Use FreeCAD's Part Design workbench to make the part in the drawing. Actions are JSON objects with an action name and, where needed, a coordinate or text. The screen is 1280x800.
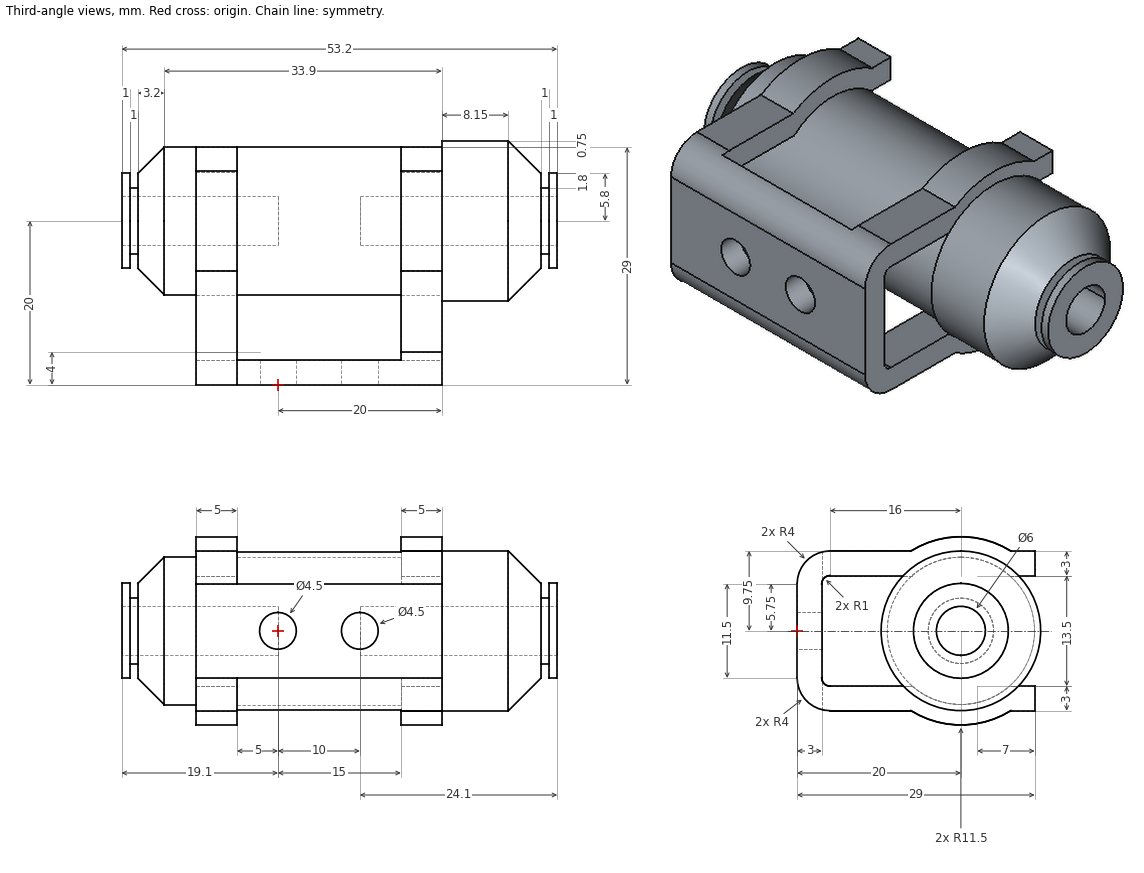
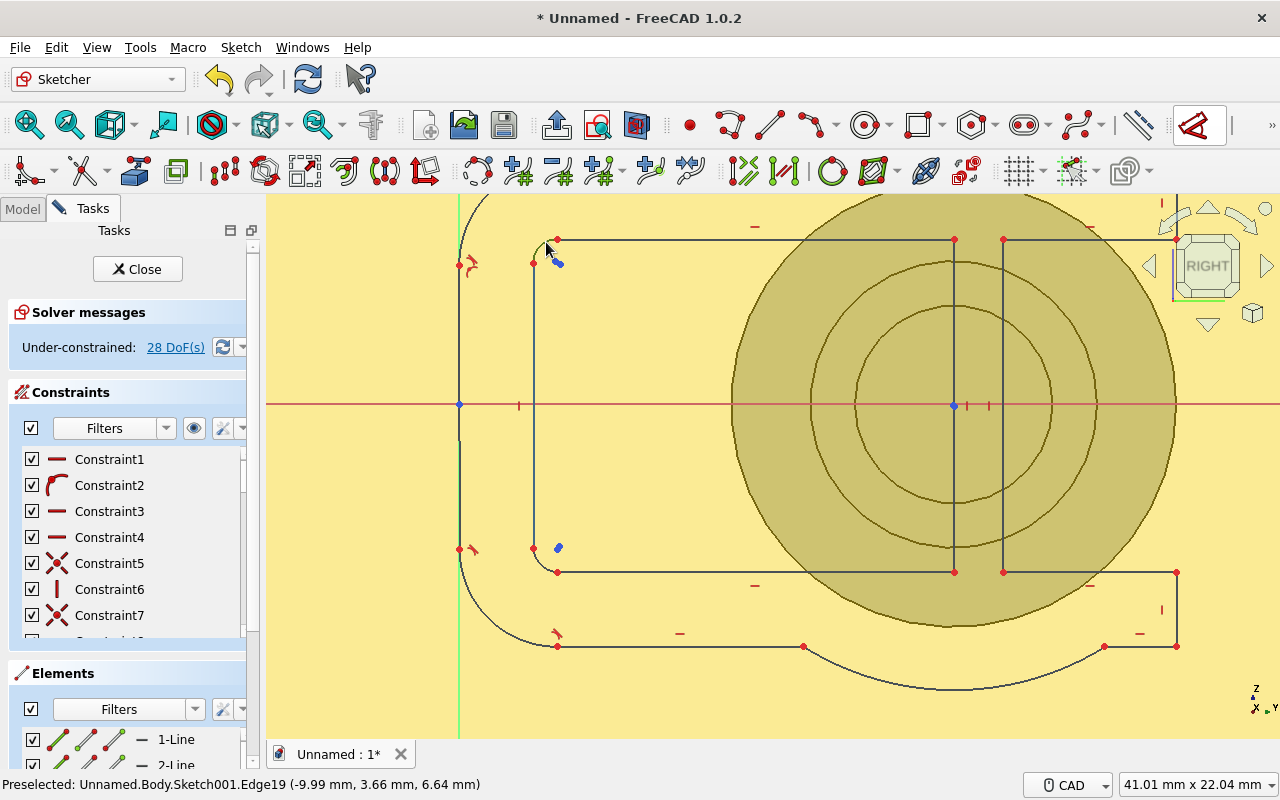
{"action": "key", "text": "t"}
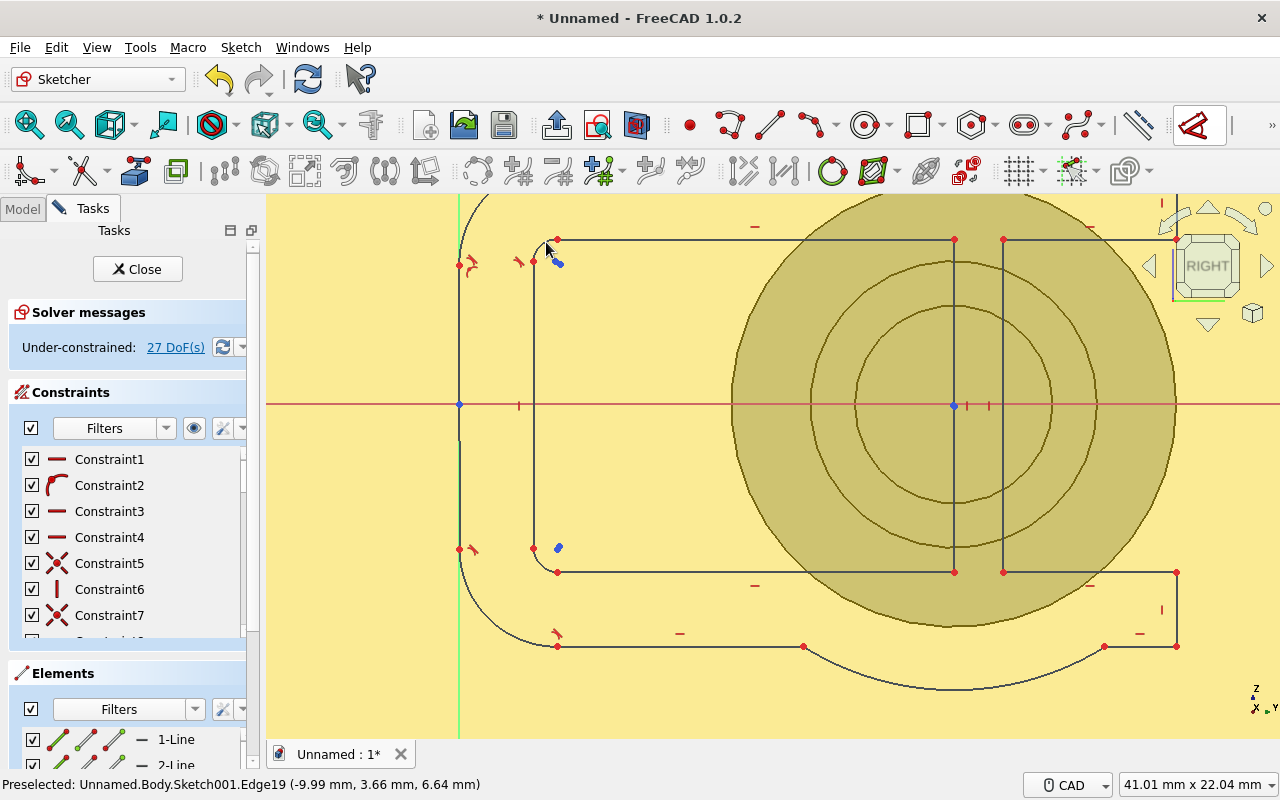
{"action": "left_click", "coordinate": [534, 462]}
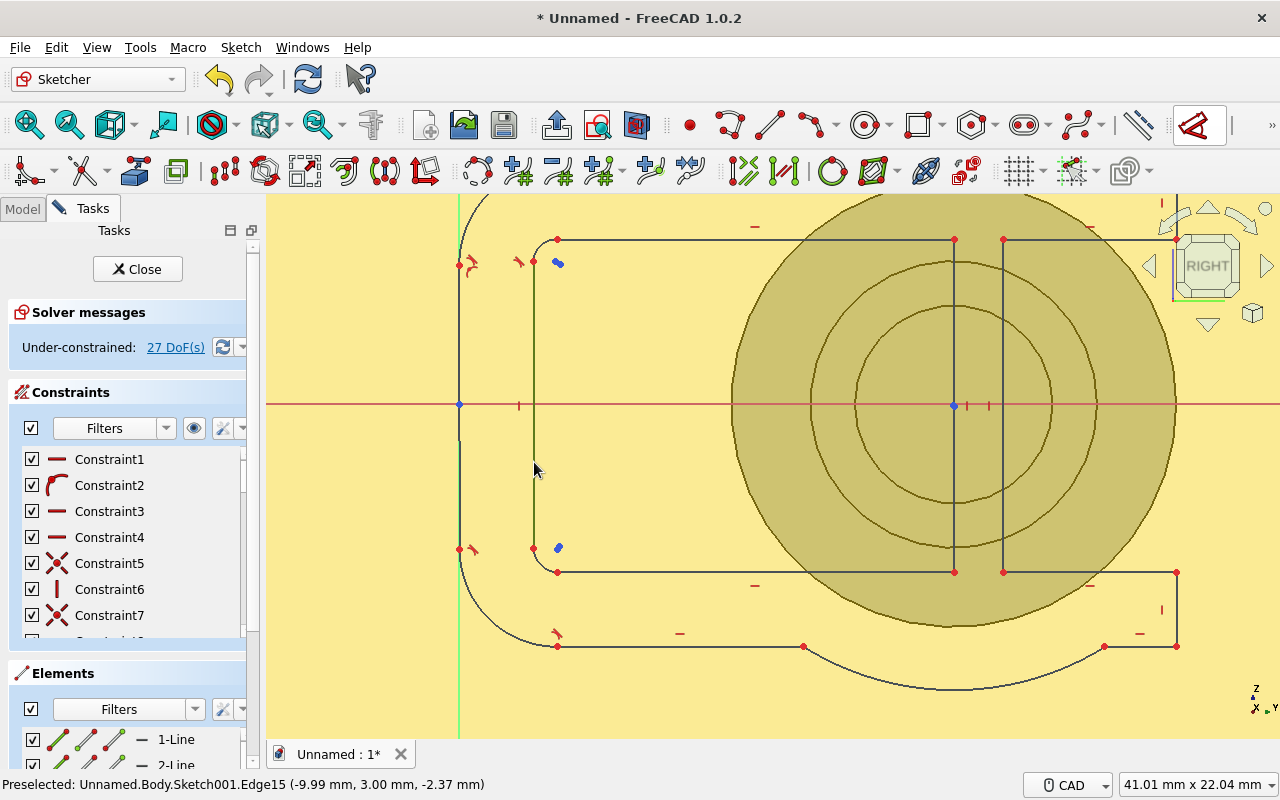
{"action": "scroll", "coordinate": [537, 559], "scroll_direction": "up", "scroll_amount": 2}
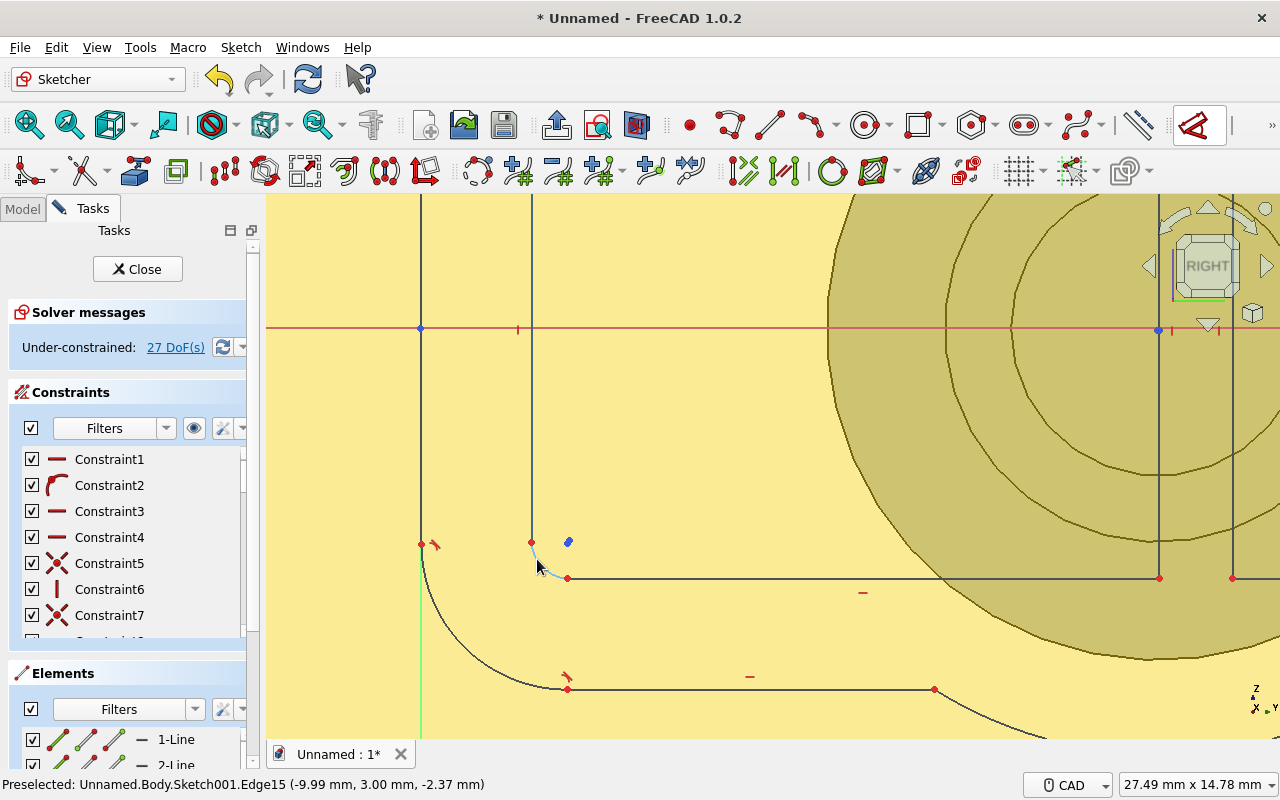
{"action": "left_click", "coordinate": [536, 559]}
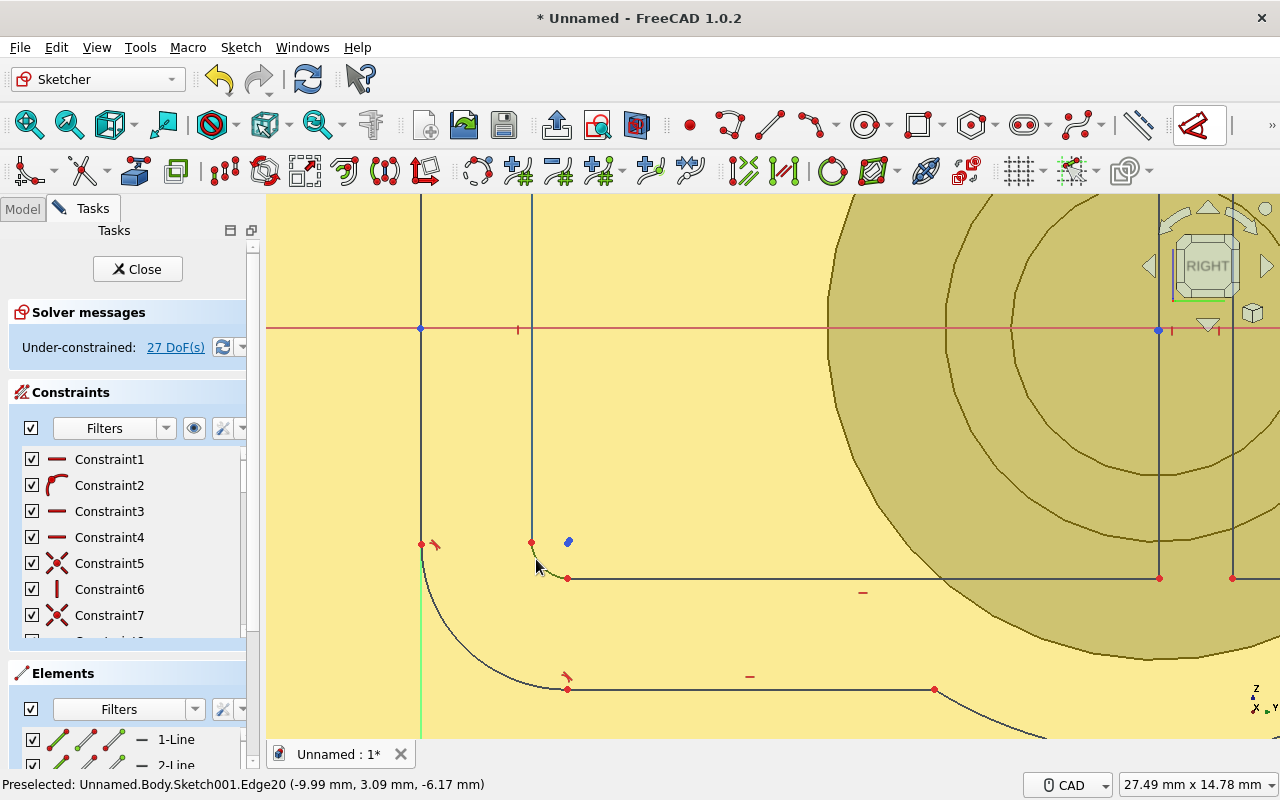
{"action": "key", "text": "t"}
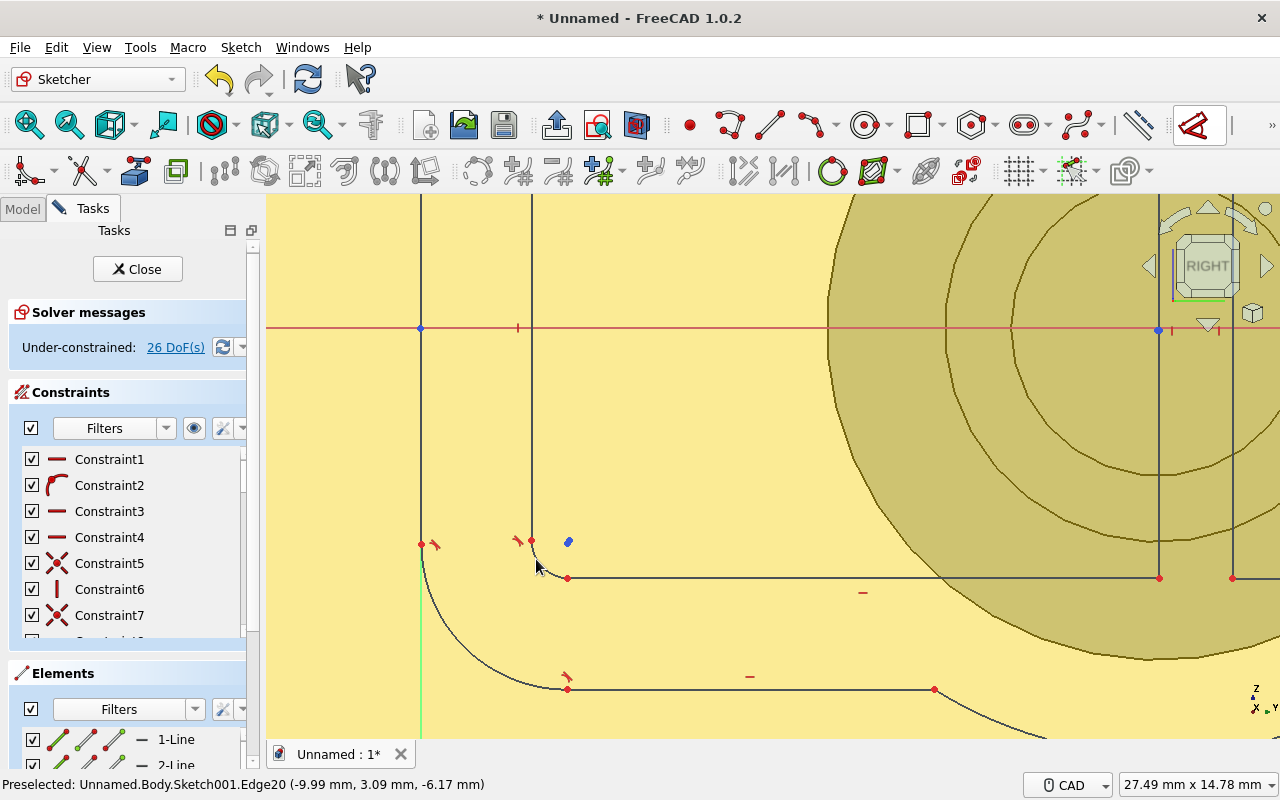
{"action": "scroll", "coordinate": [500, 579], "scroll_direction": "down", "scroll_amount": 4}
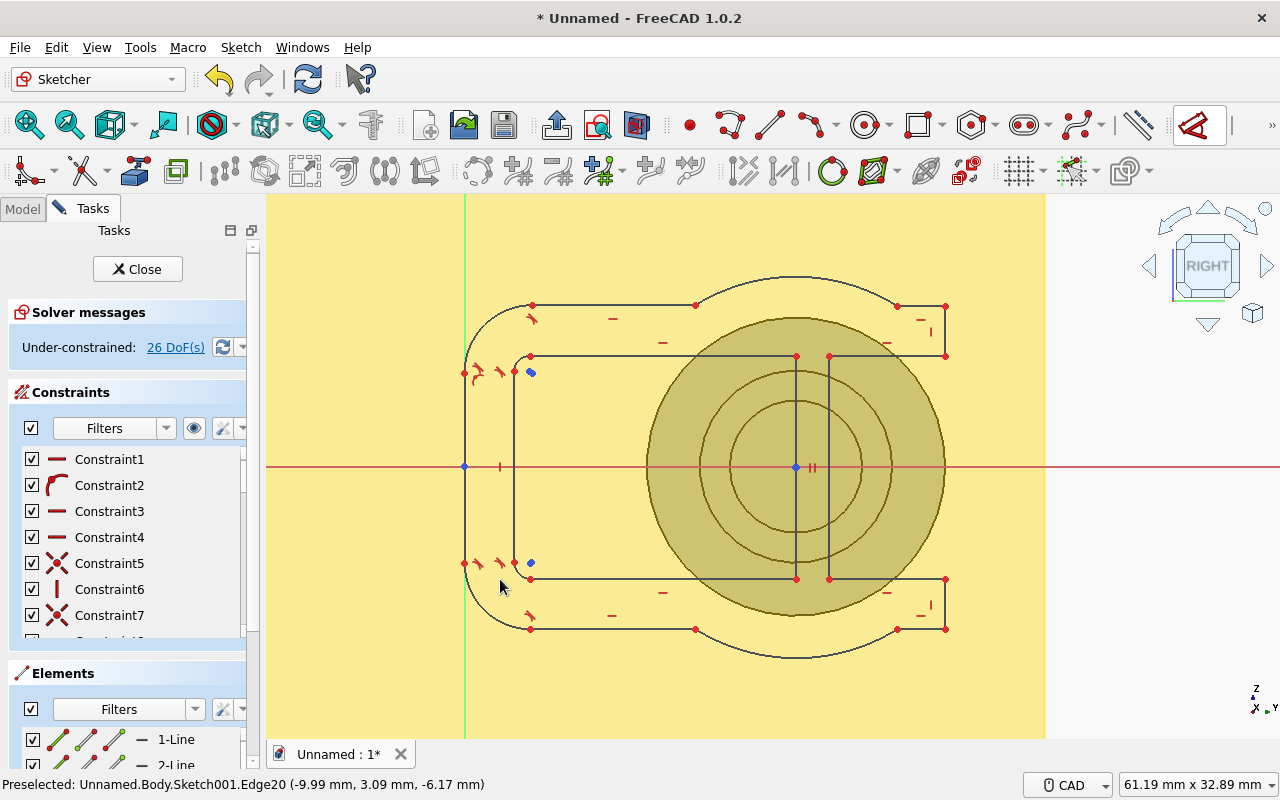
{"action": "left_click", "coordinate": [610, 356]}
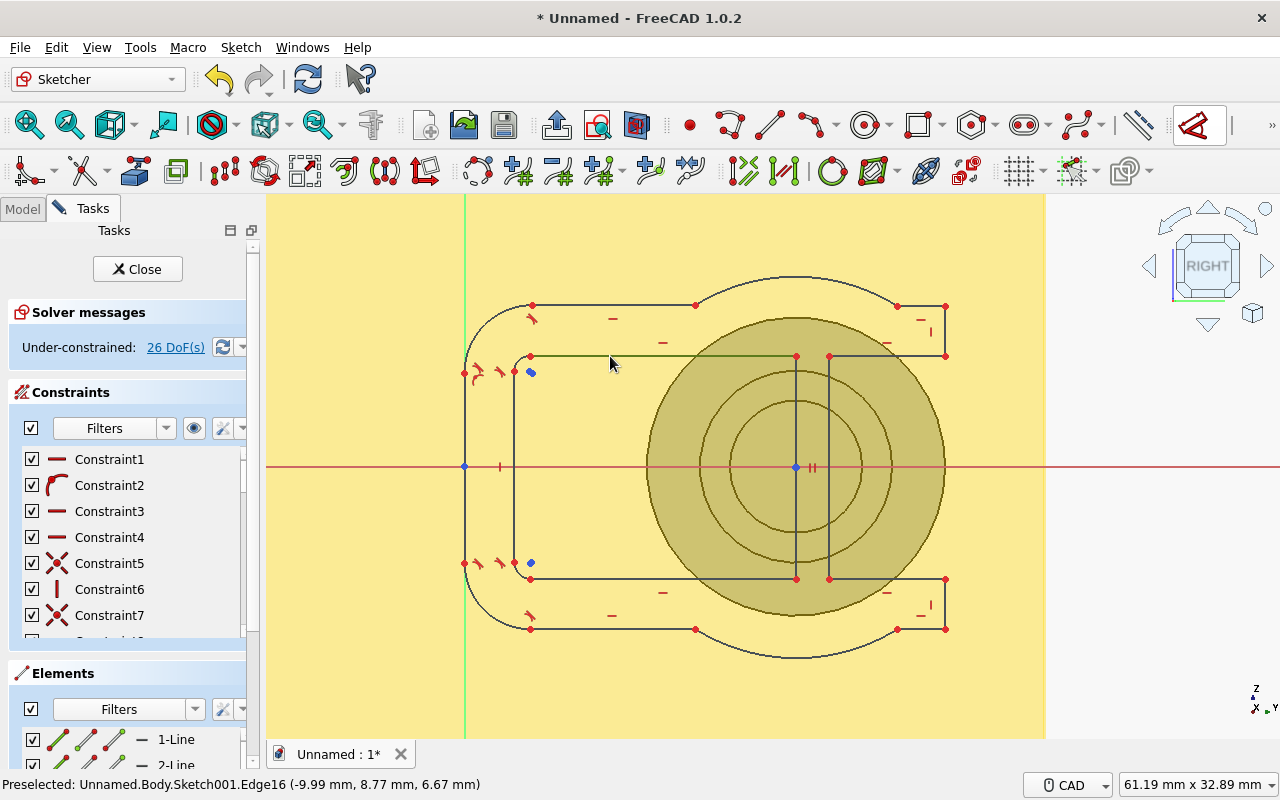
{"action": "left_click", "coordinate": [519, 360]}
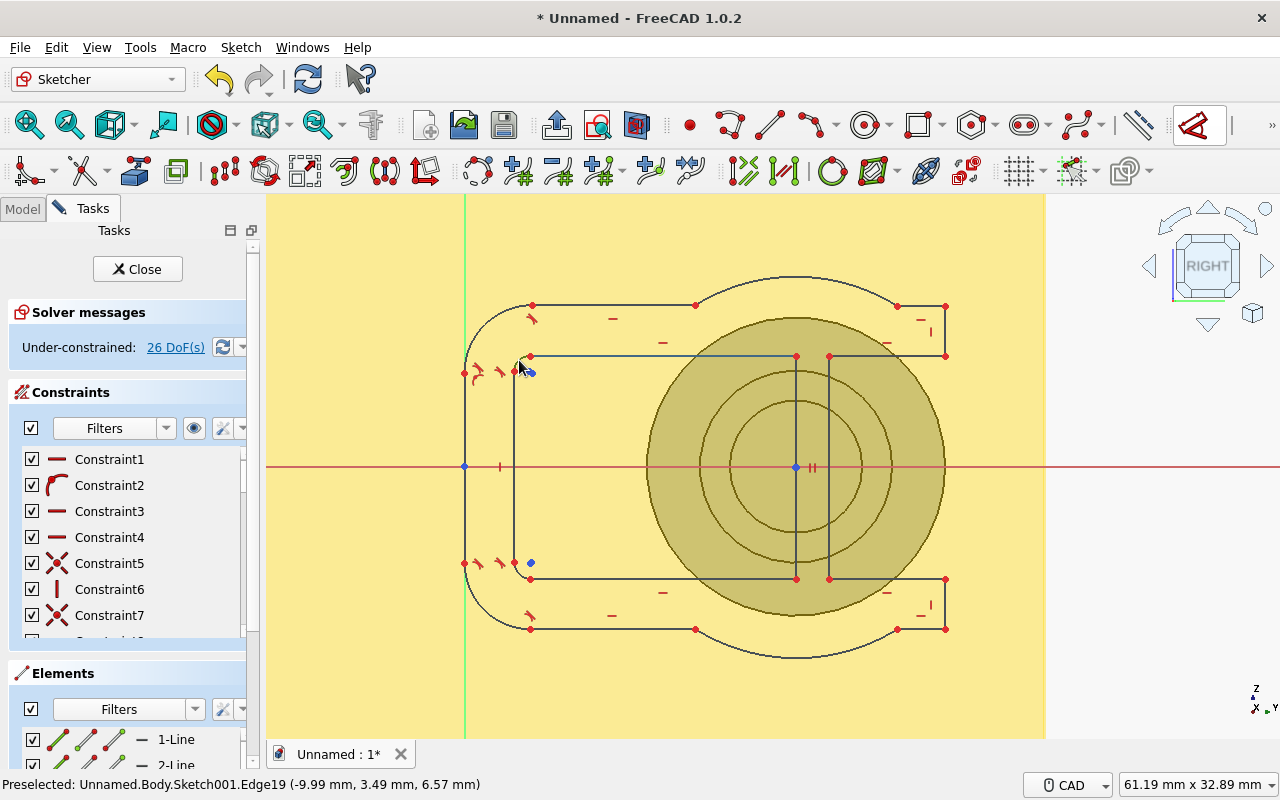
{"action": "key", "text": "t"}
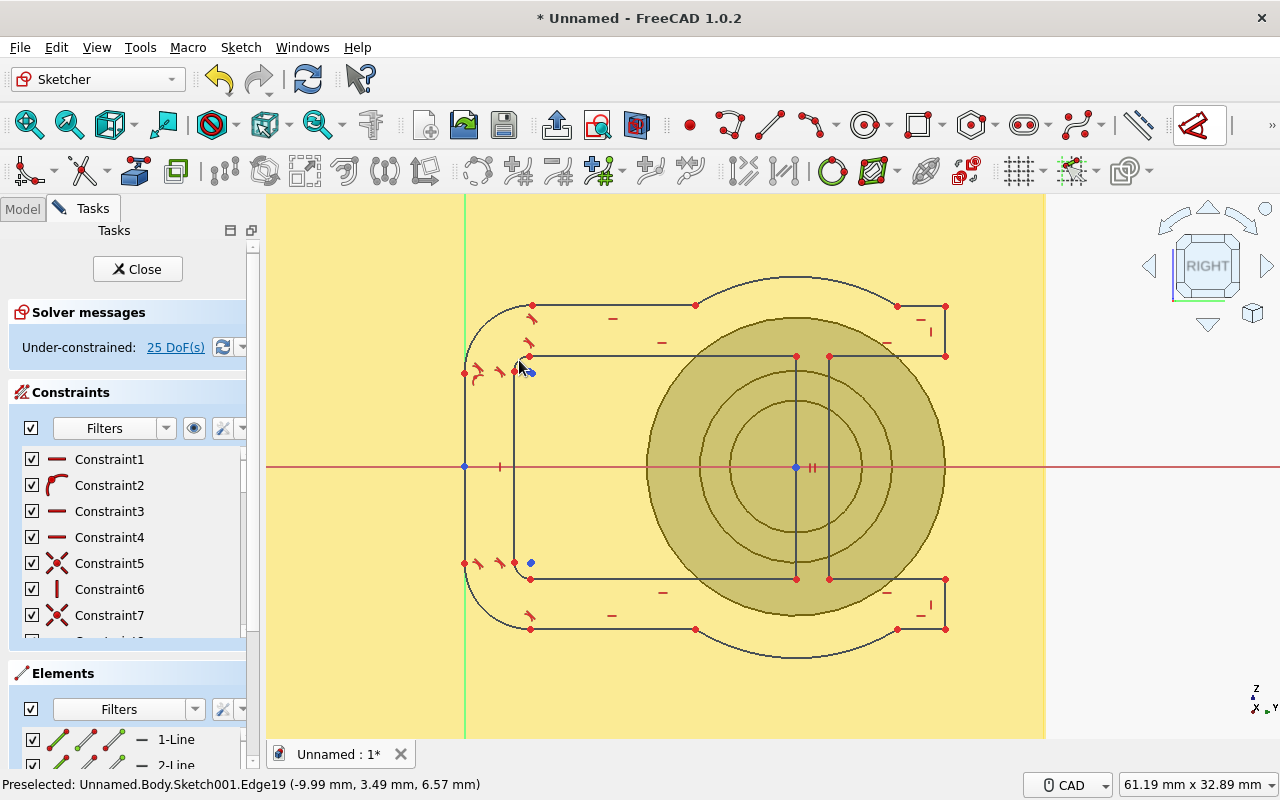
{"action": "left_click", "coordinate": [717, 579]}